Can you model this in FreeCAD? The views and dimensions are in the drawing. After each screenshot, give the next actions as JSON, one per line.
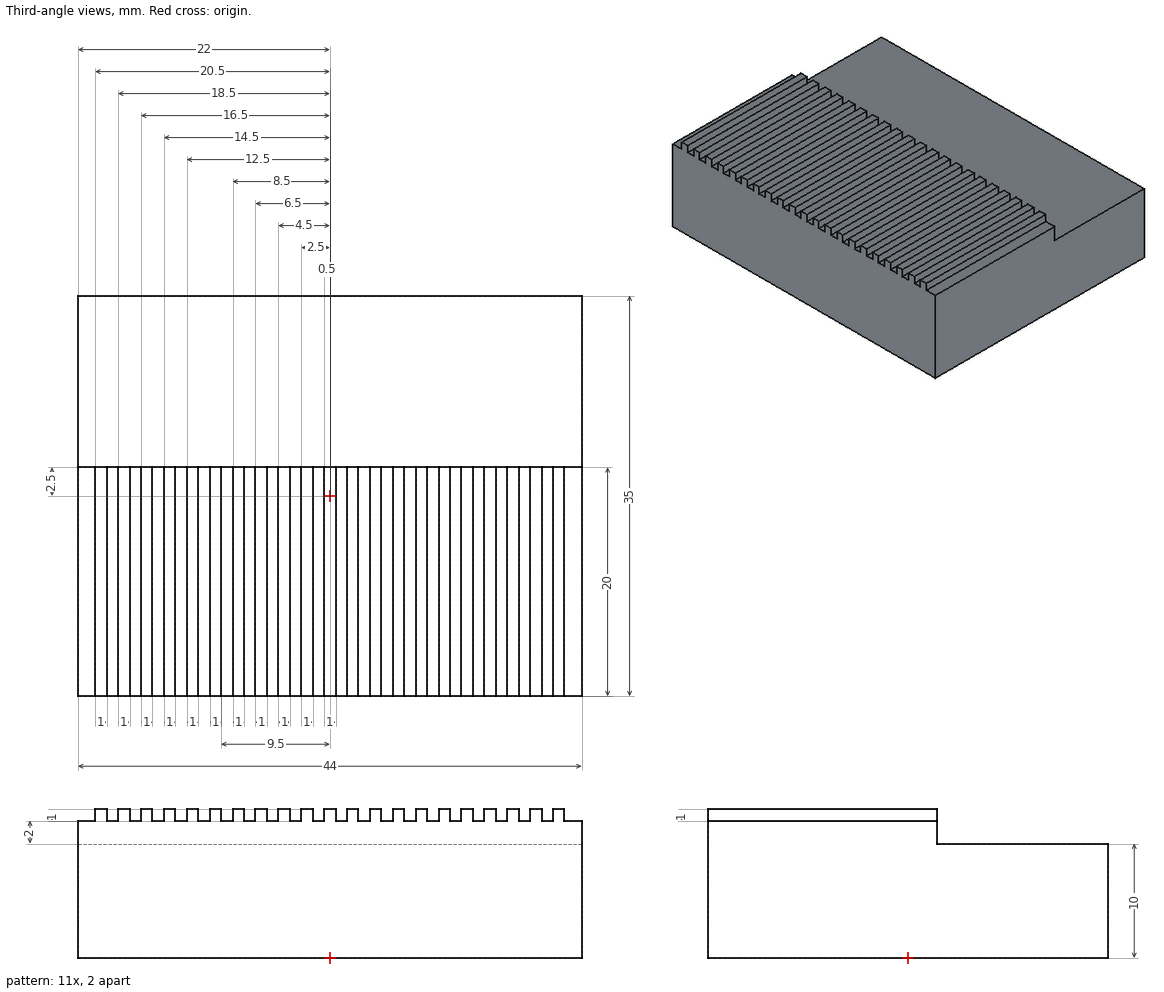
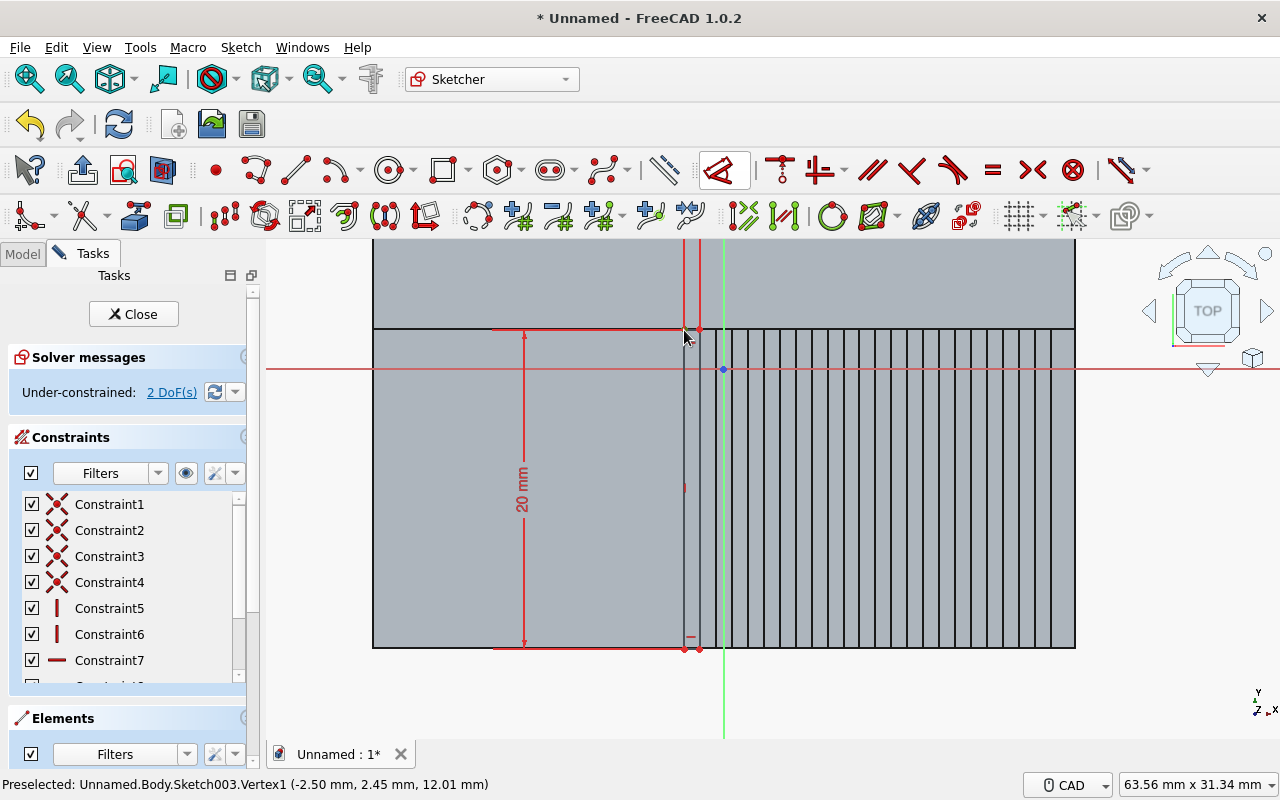
{"action": "left_click", "coordinate": [744, 170]}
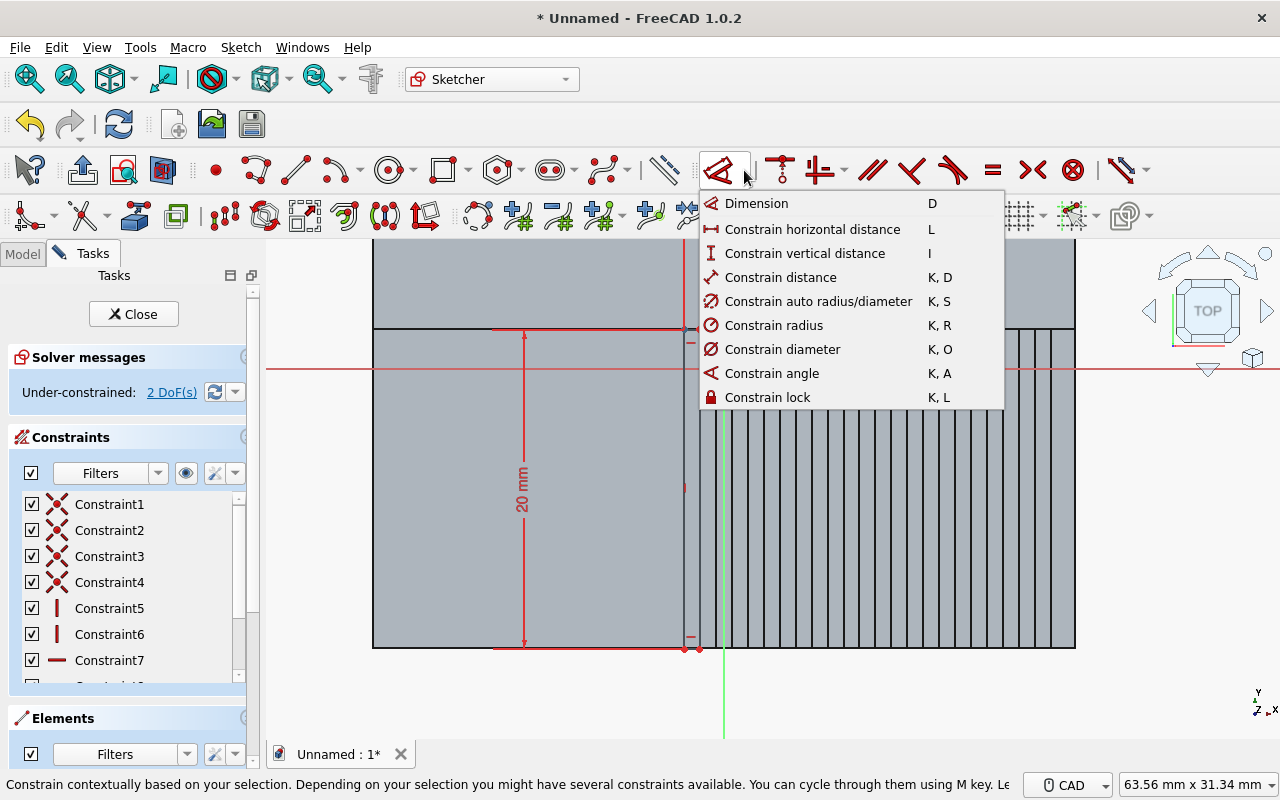
{"action": "left_click", "coordinate": [852, 229]}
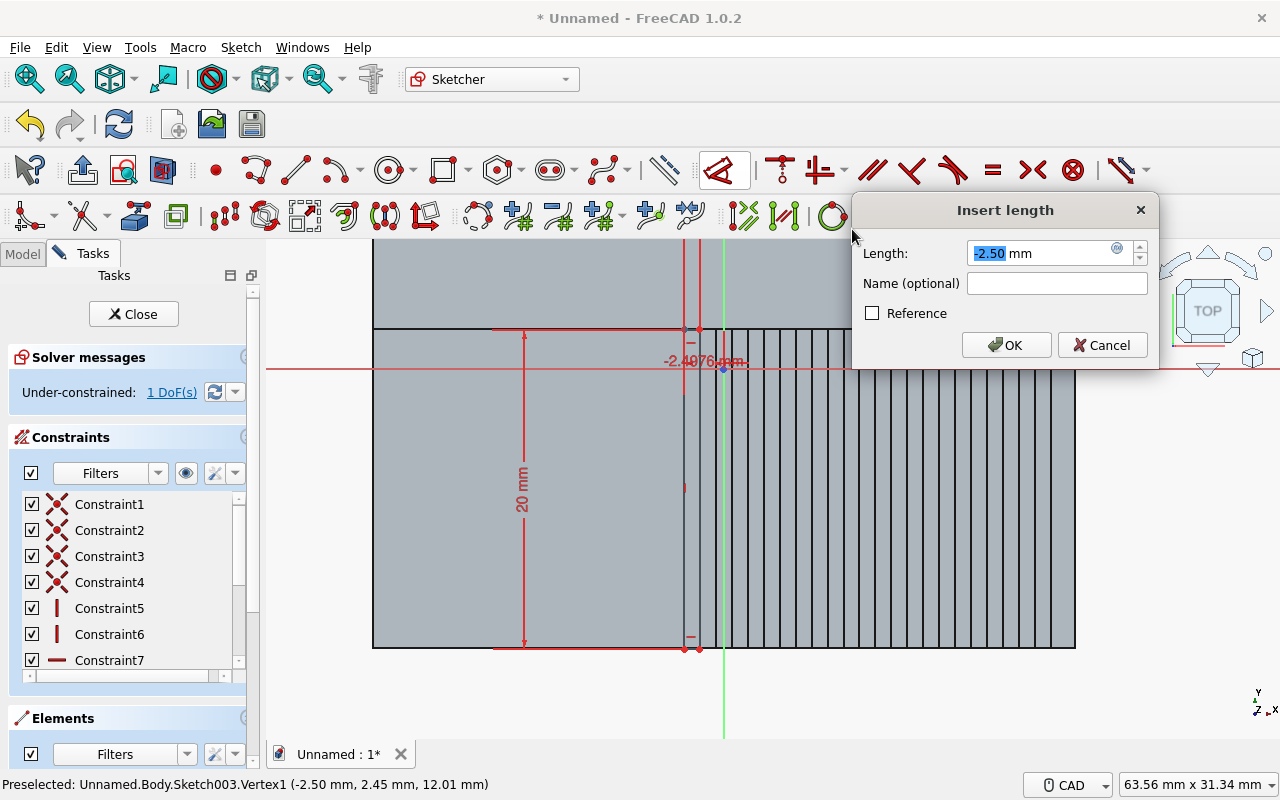
{"action": "type", "text": "-2.5"}
{"action": "key", "text": "Return"}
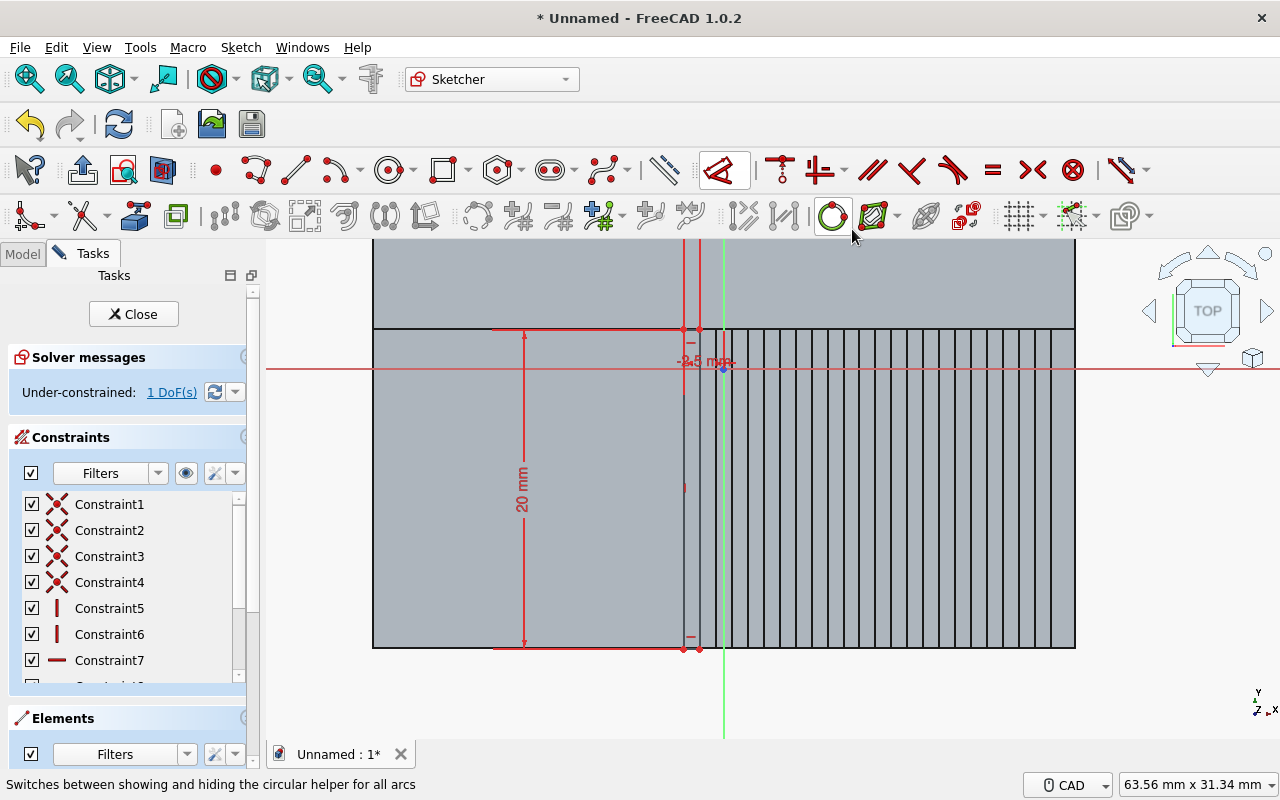
{"action": "left_click", "coordinate": [684, 330]}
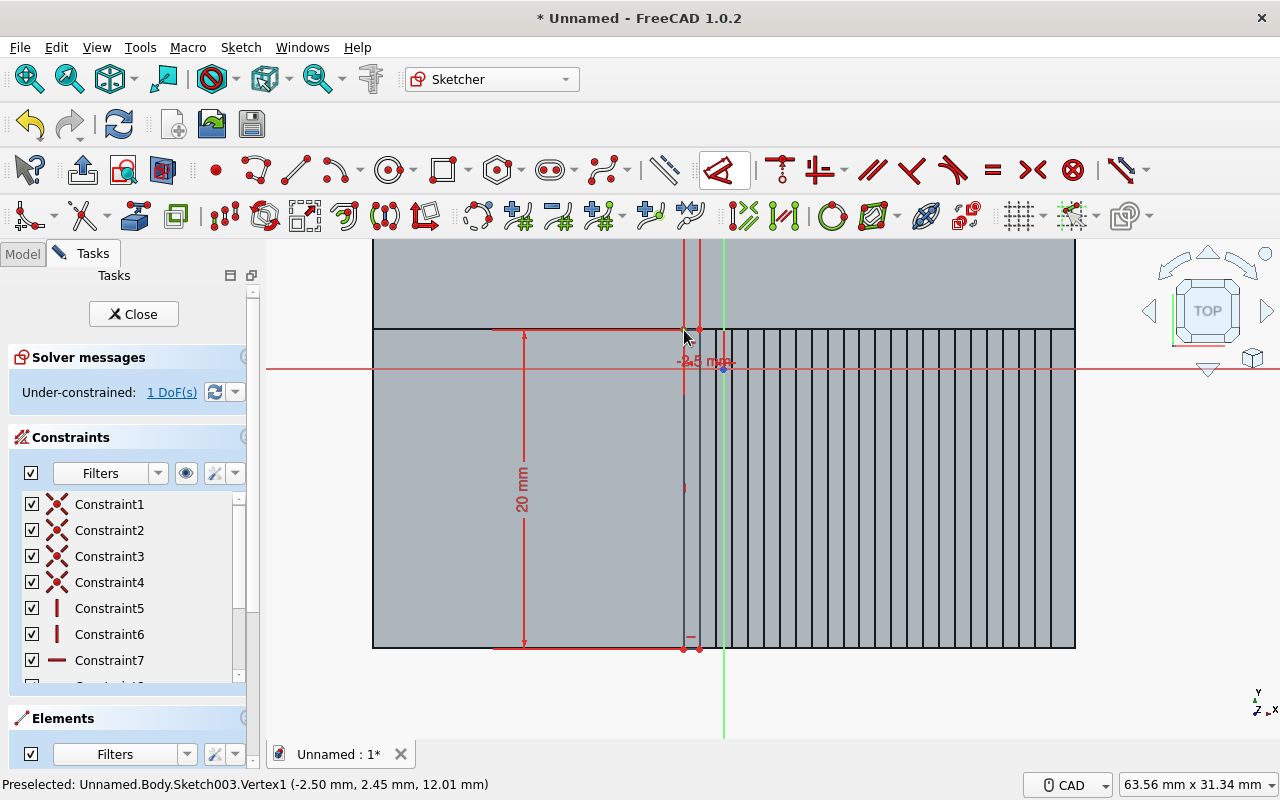
{"action": "key", "text": "i"}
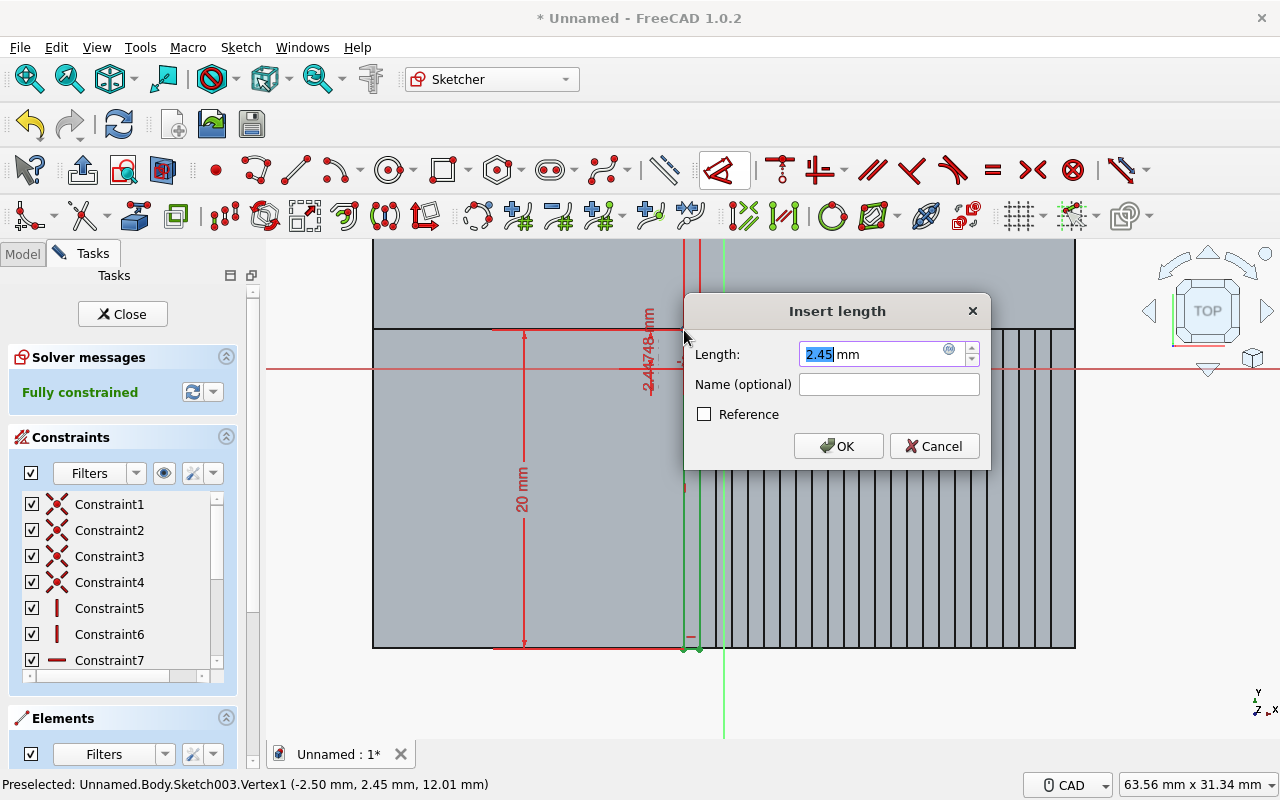
{"action": "type", "text": "2.5"}
{"action": "key", "text": "Return"}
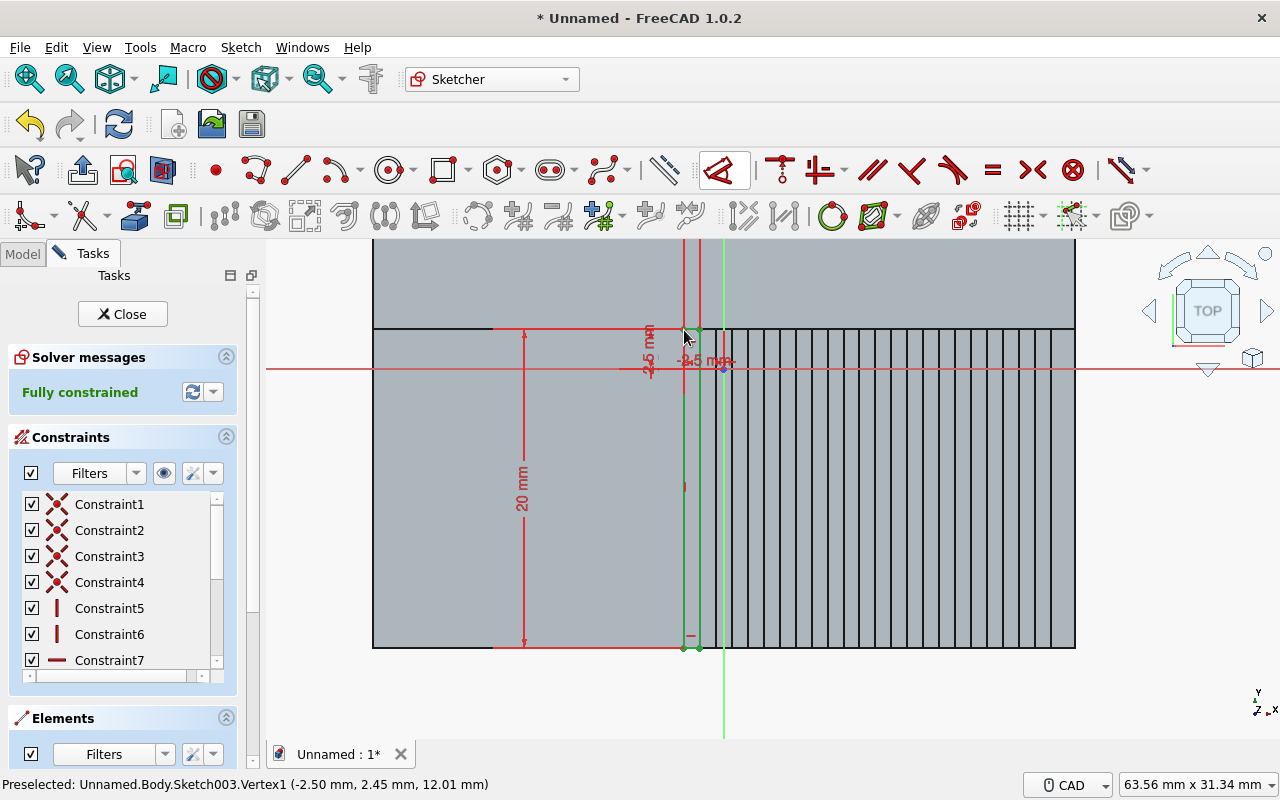
{"action": "left_click", "coordinate": [123, 314]}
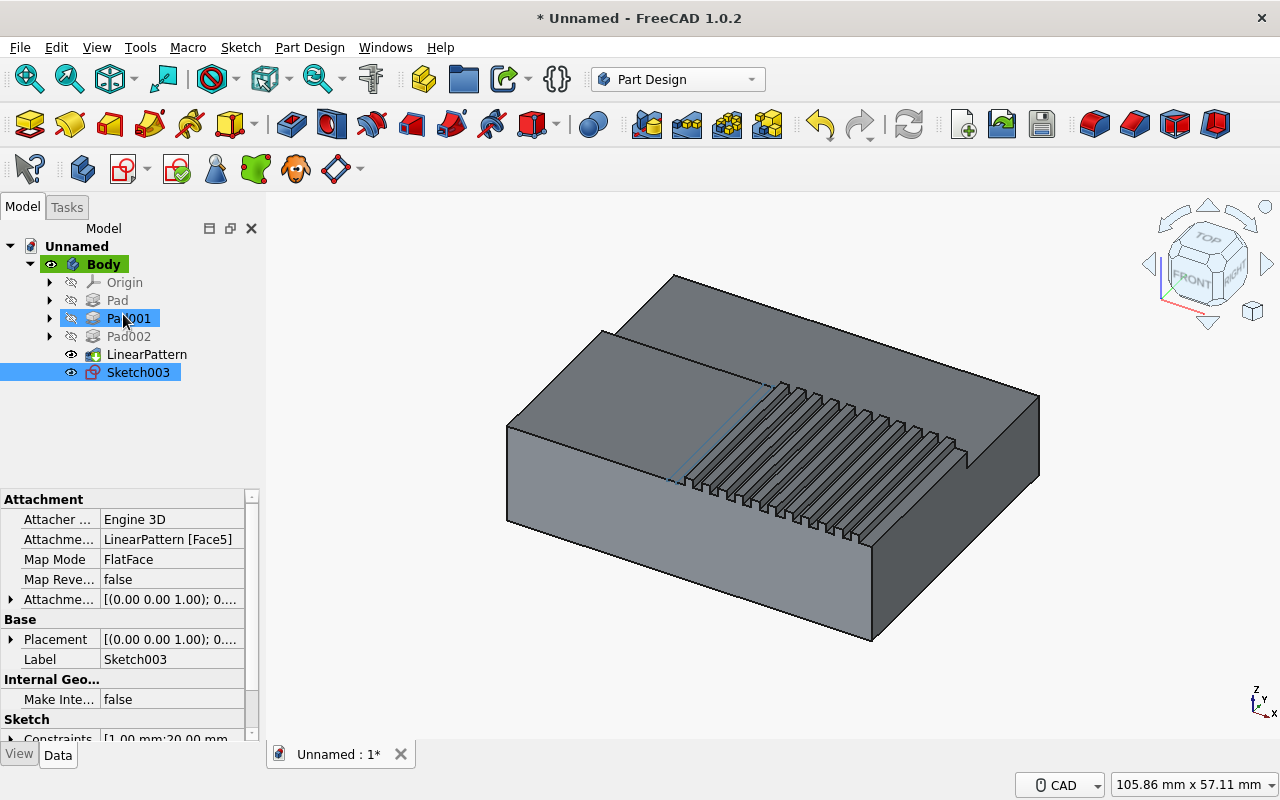
{"action": "left_click", "coordinate": [30, 124]}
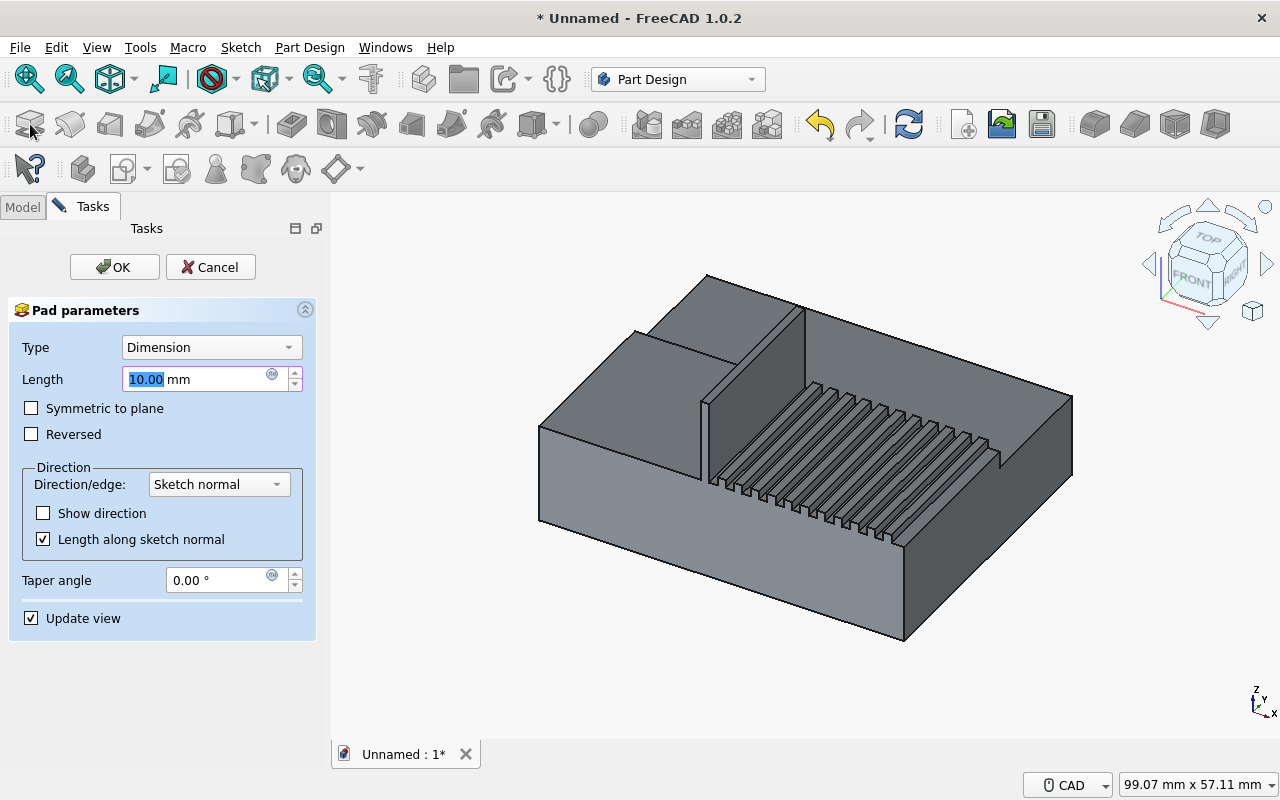
{"action": "type", "text": "1"}
{"action": "key", "text": "Tab"}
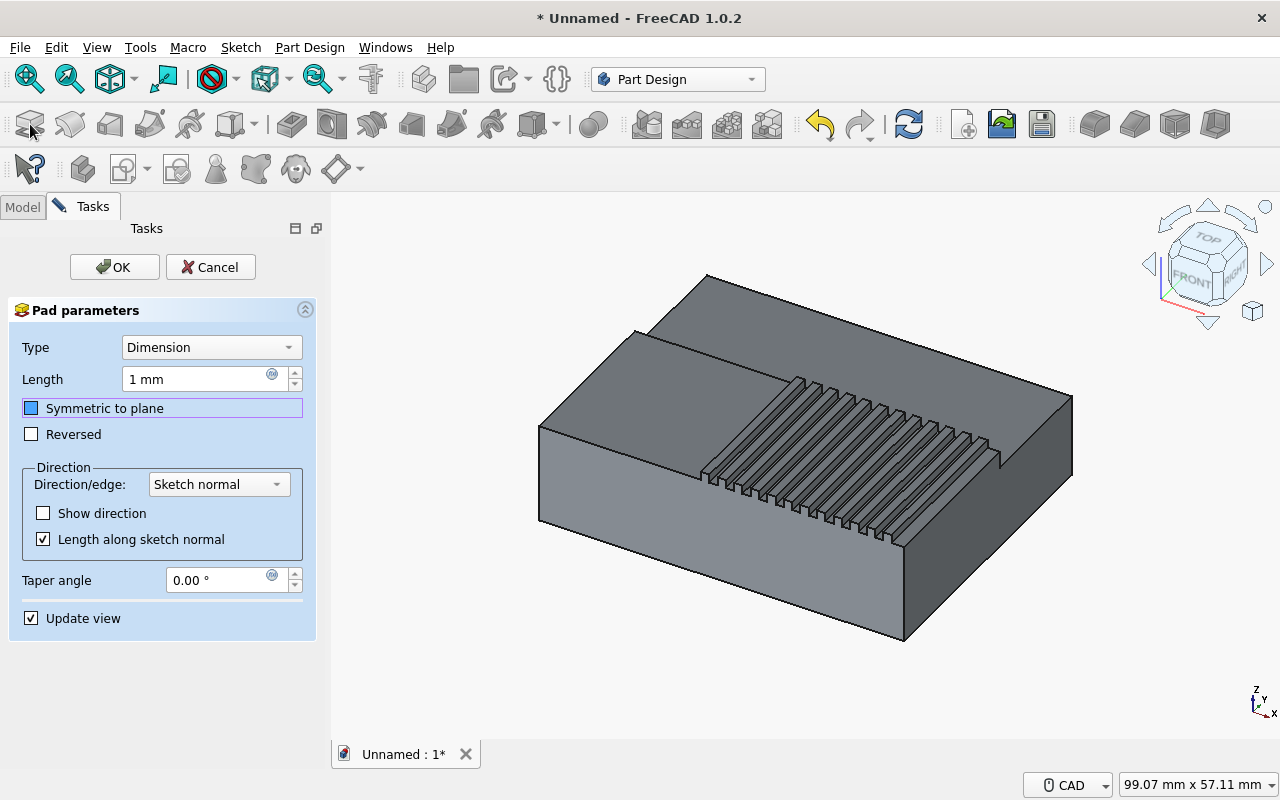
{"action": "left_click", "coordinate": [115, 267]}